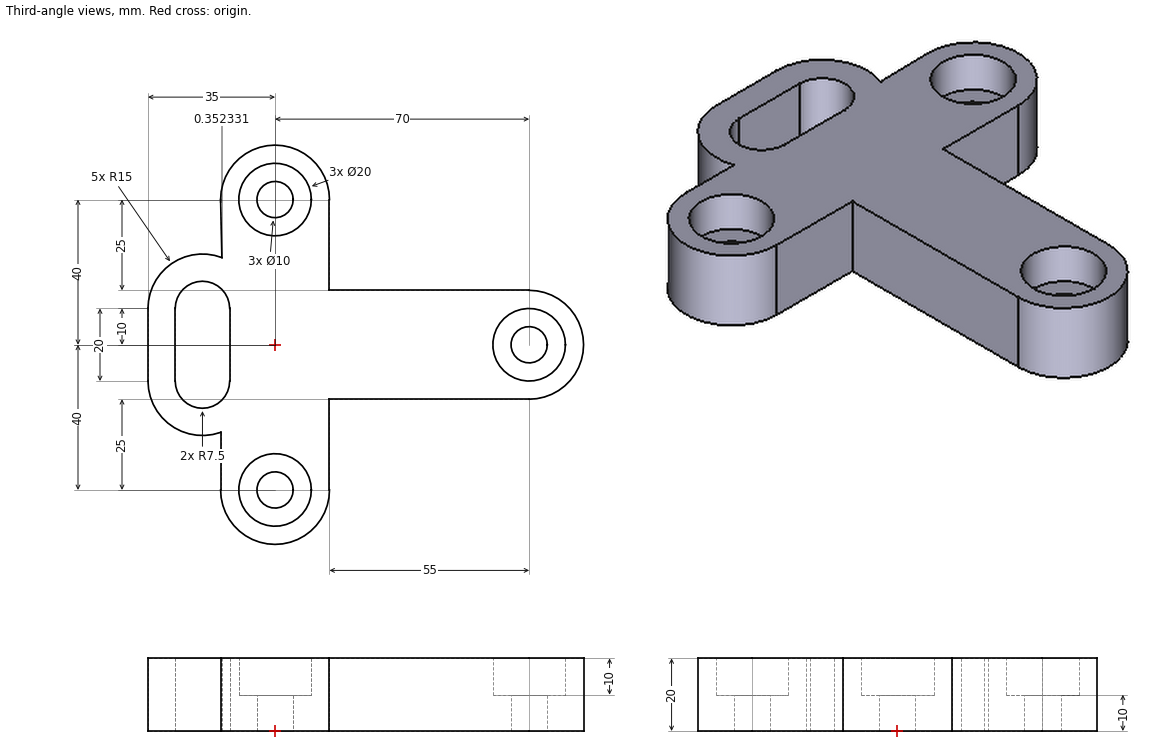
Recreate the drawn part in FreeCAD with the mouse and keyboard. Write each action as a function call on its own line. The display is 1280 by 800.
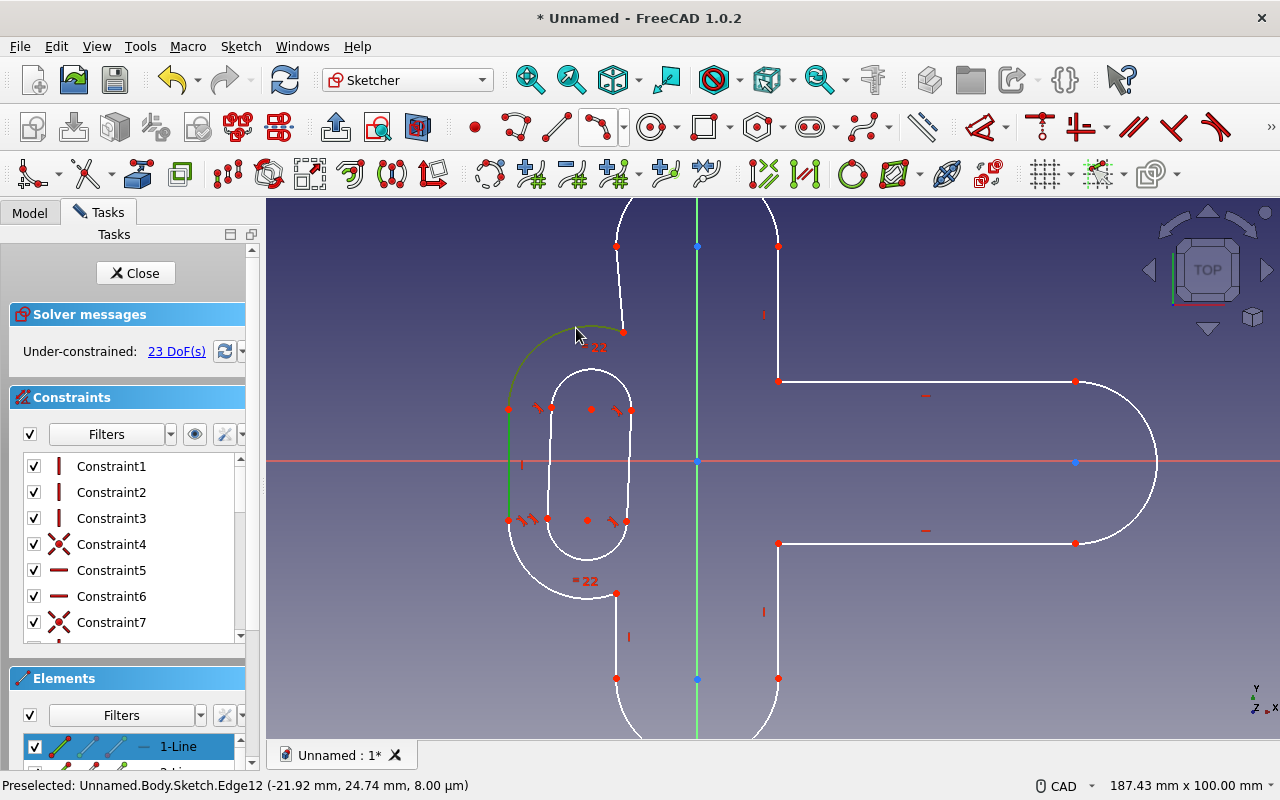
click(1216, 128)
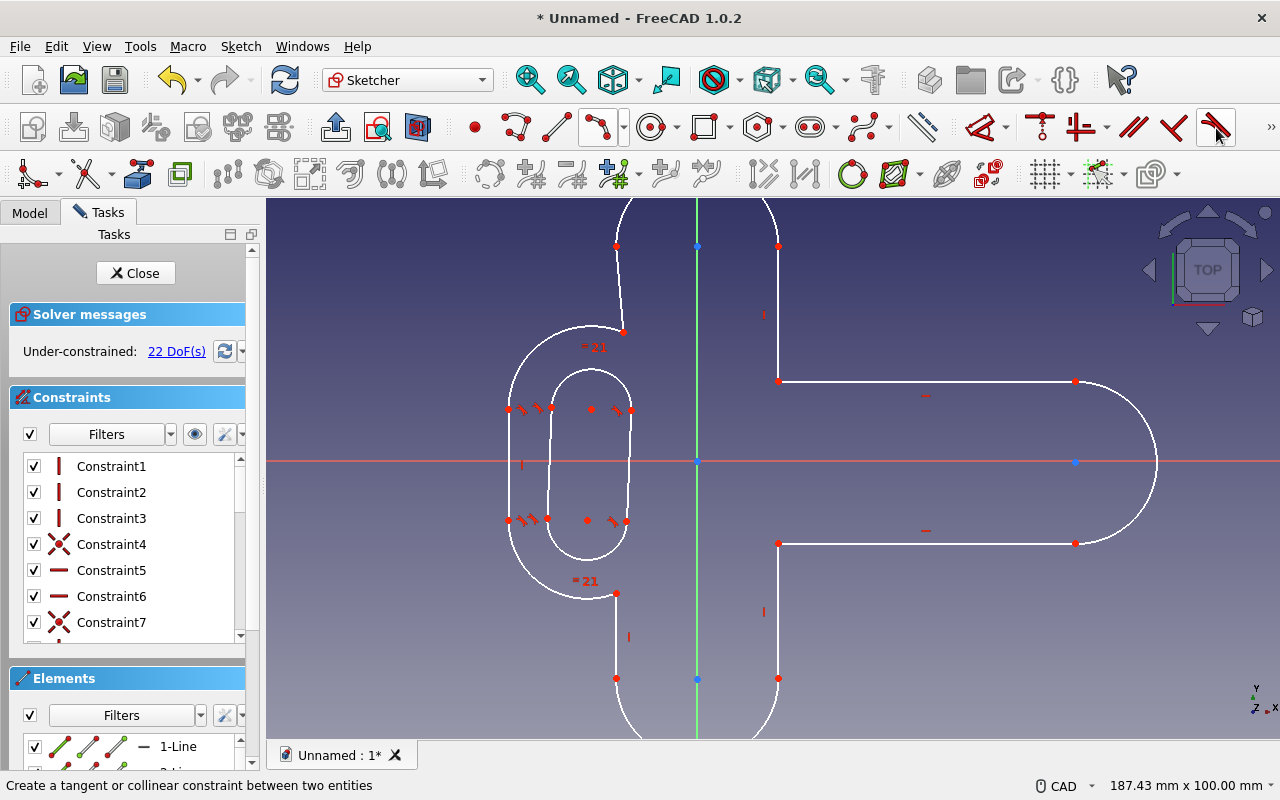
click(616, 619)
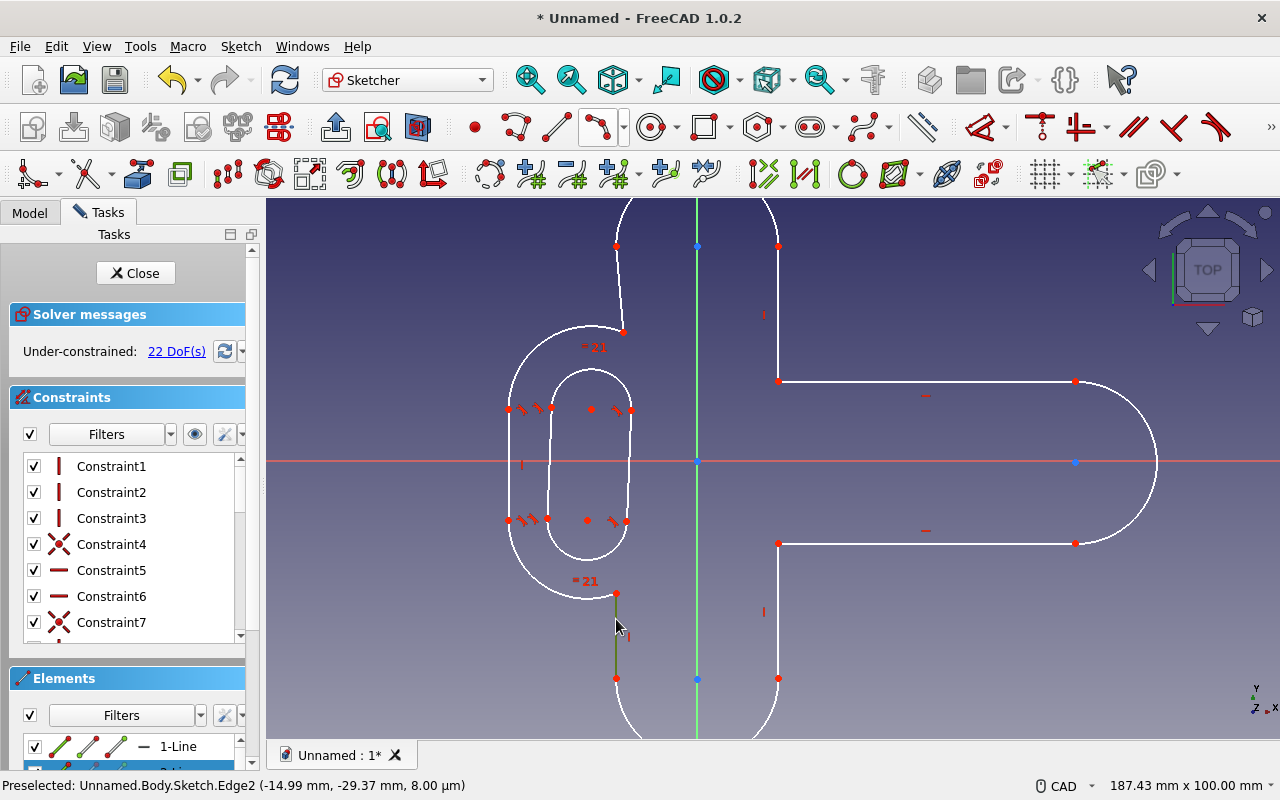
scroll(549, 478, down, 3)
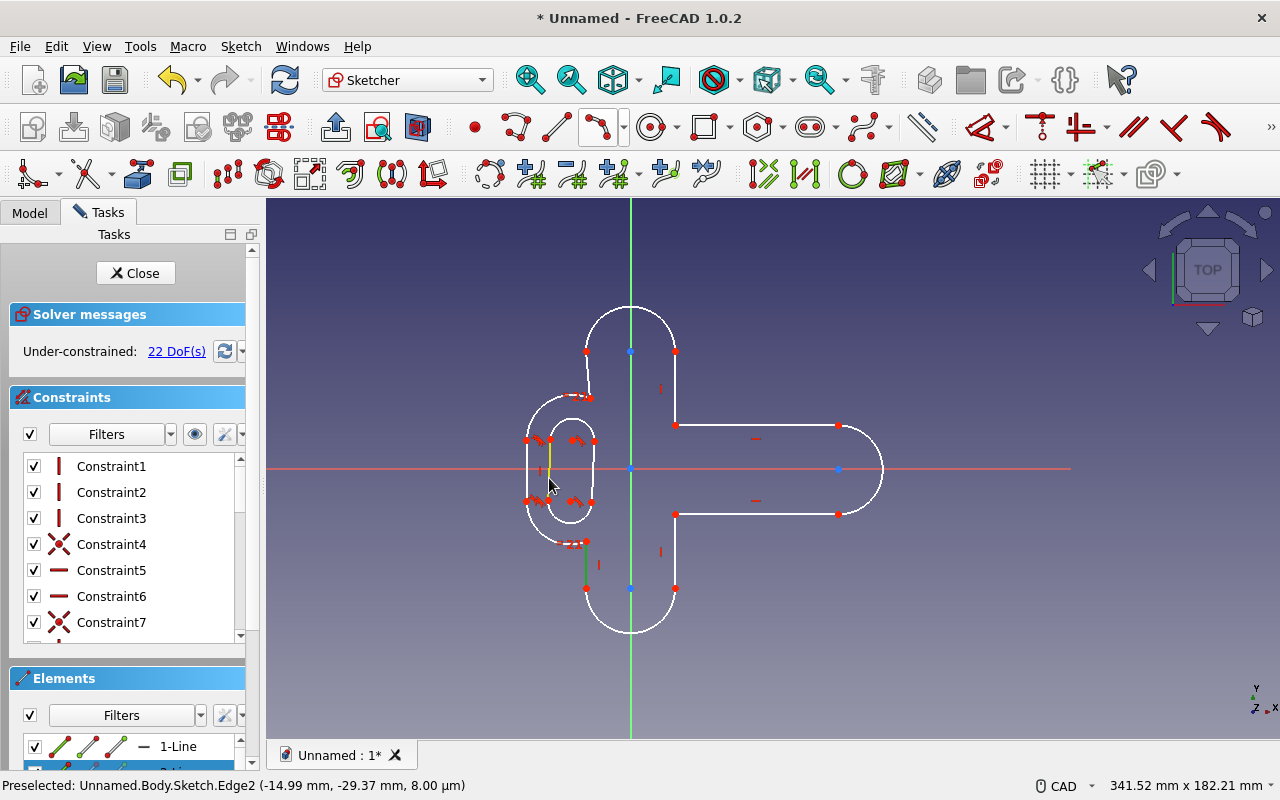
click(604, 625)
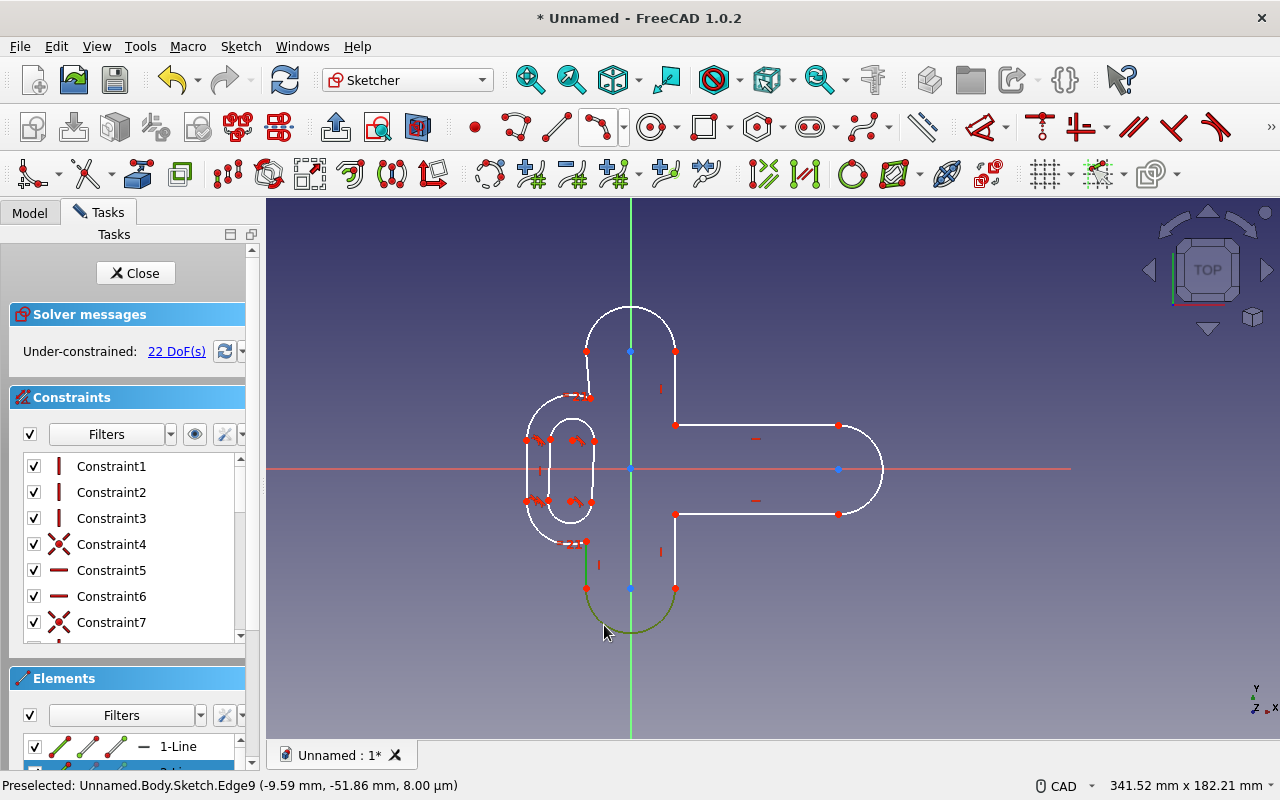
click(1216, 128)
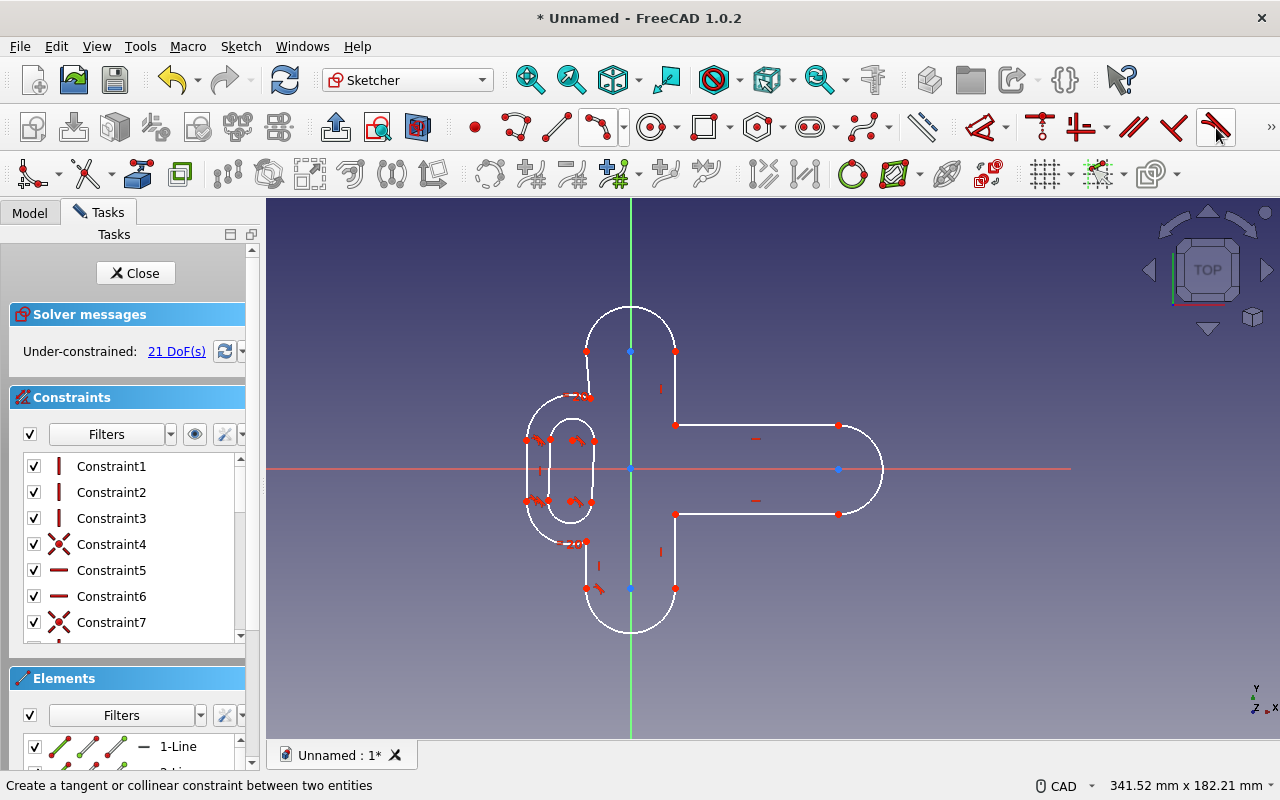
click(675, 566)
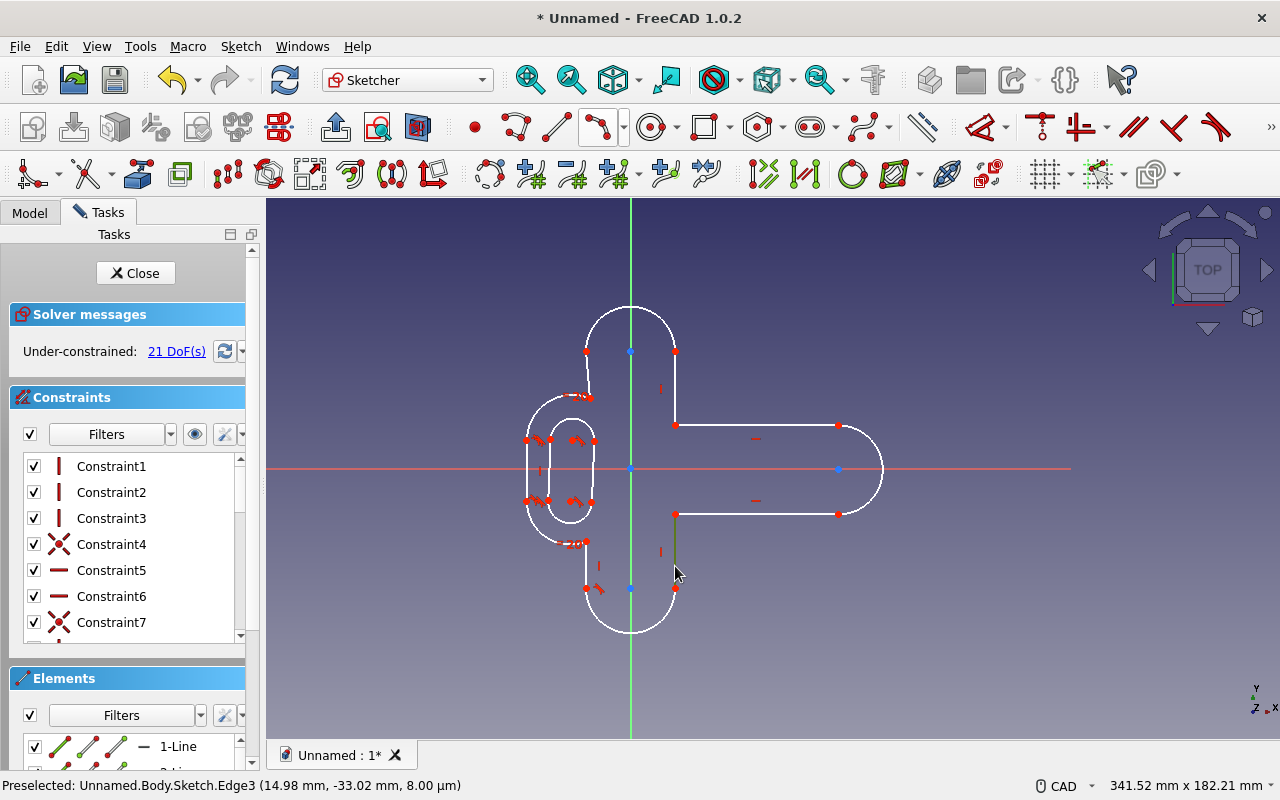
click(604, 625)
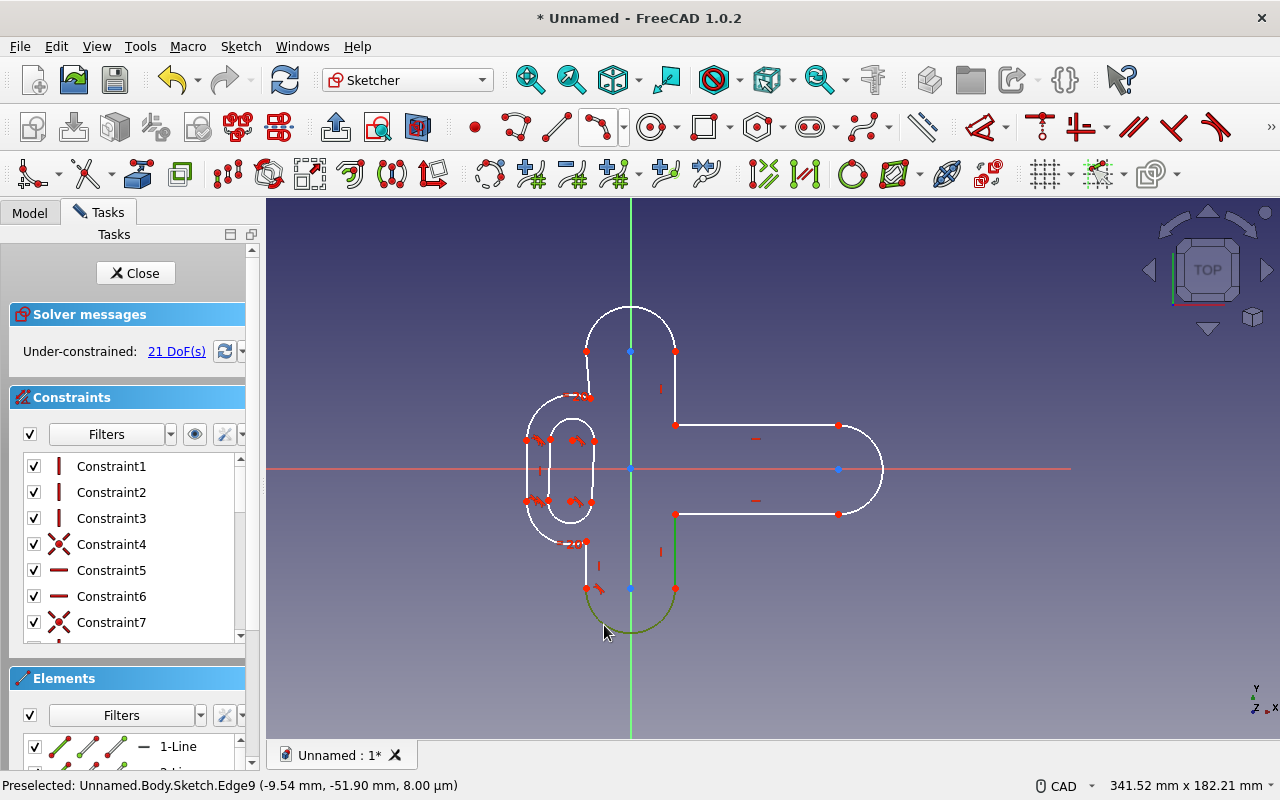
click(1216, 128)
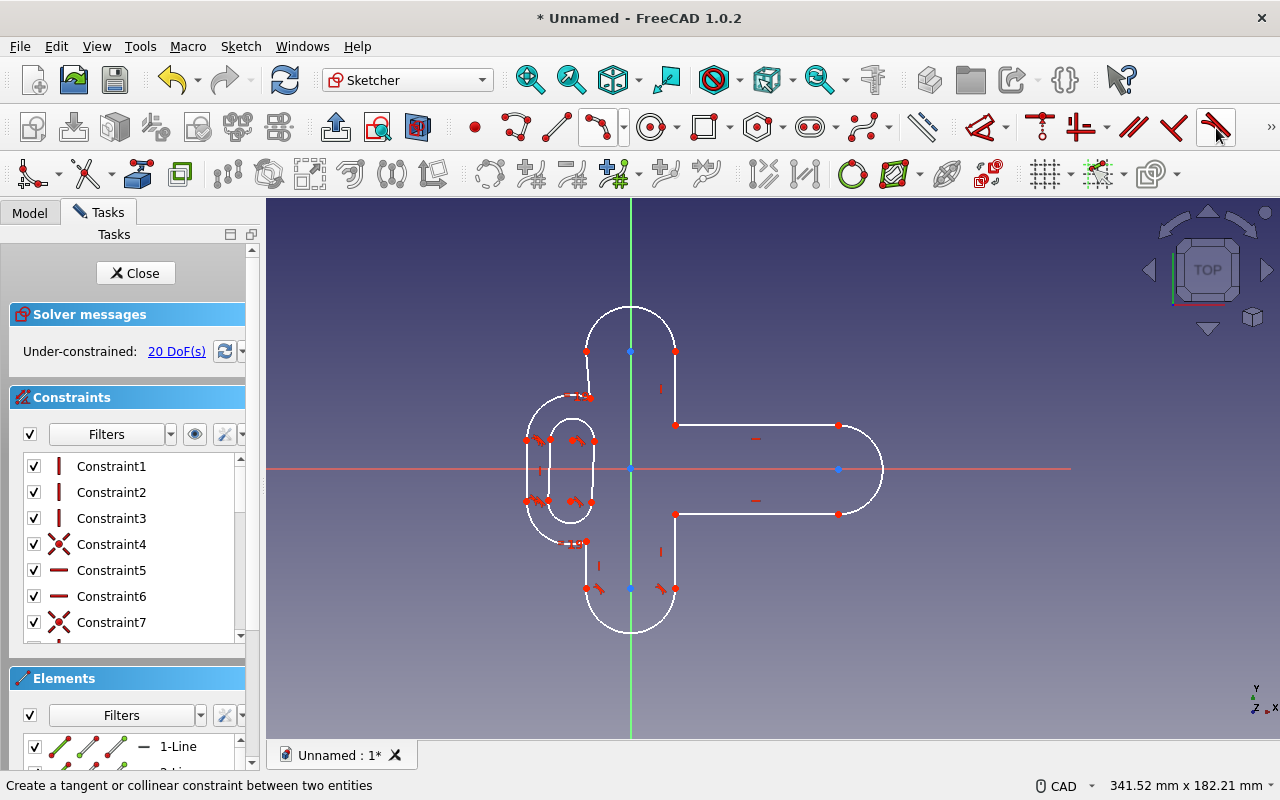
click(724, 514)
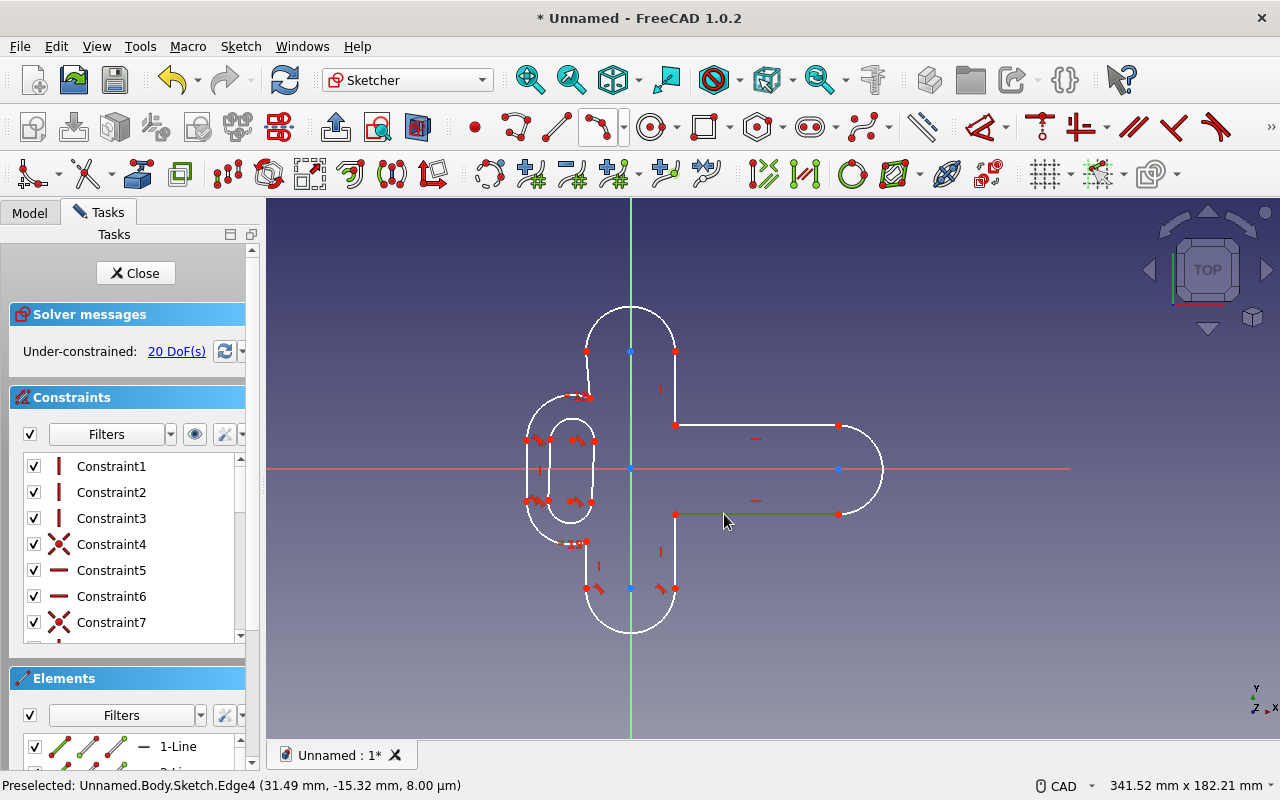
click(874, 496)